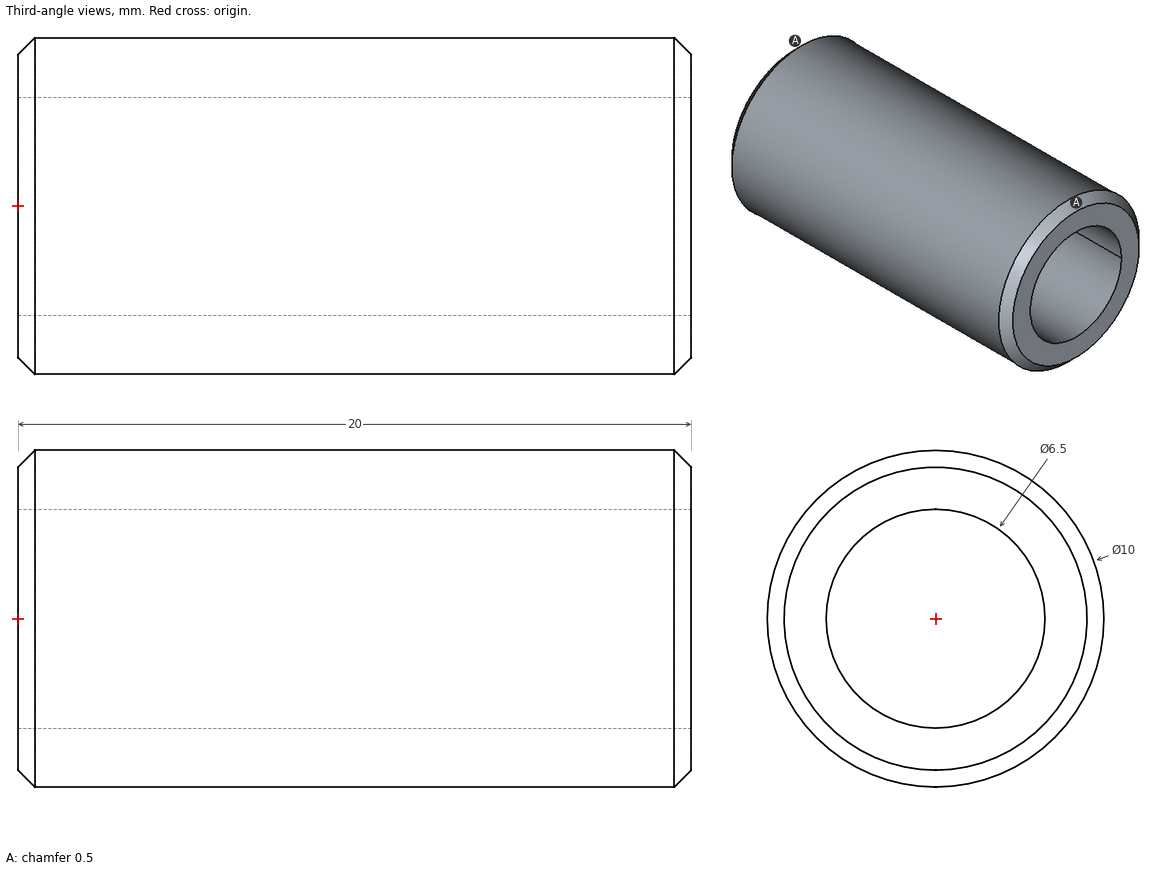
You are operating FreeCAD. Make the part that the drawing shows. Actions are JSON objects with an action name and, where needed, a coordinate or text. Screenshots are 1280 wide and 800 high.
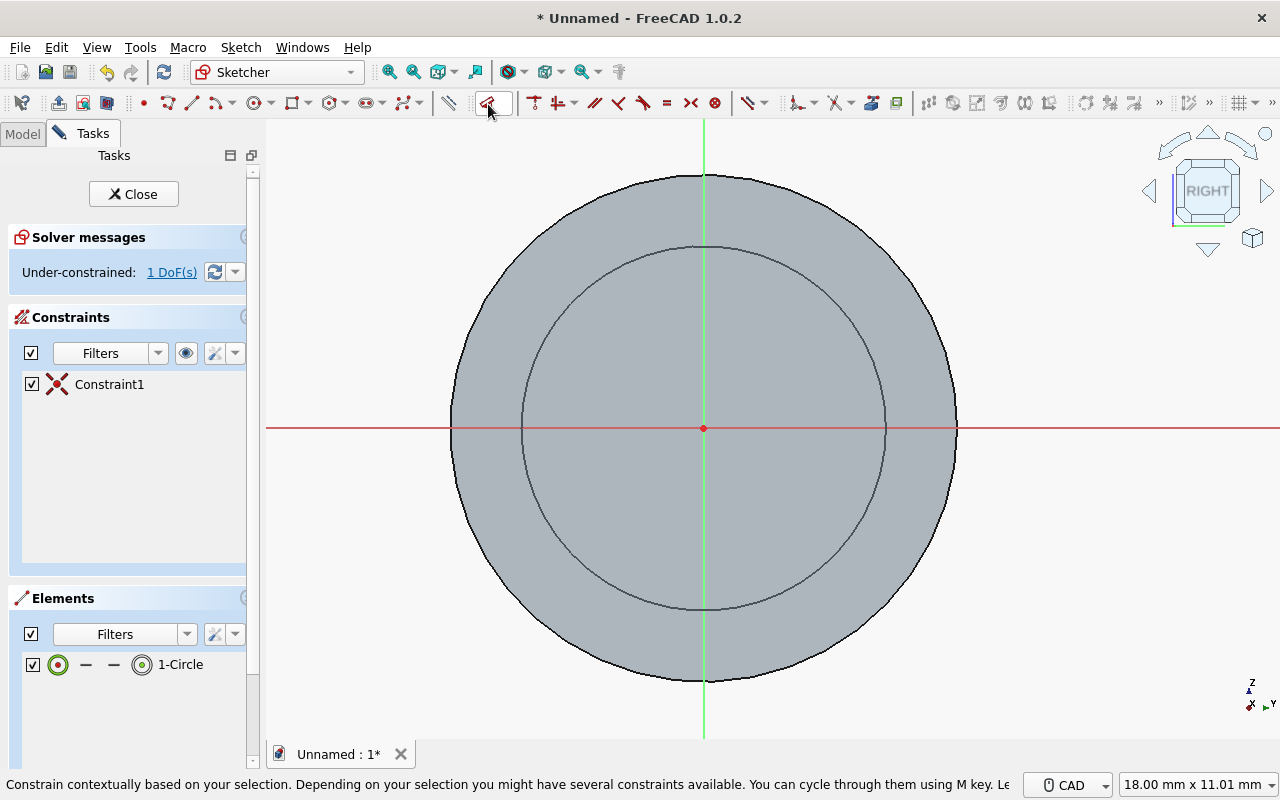
{"action": "left_click", "coordinate": [832, 299]}
{"action": "left_click", "coordinate": [855, 276]}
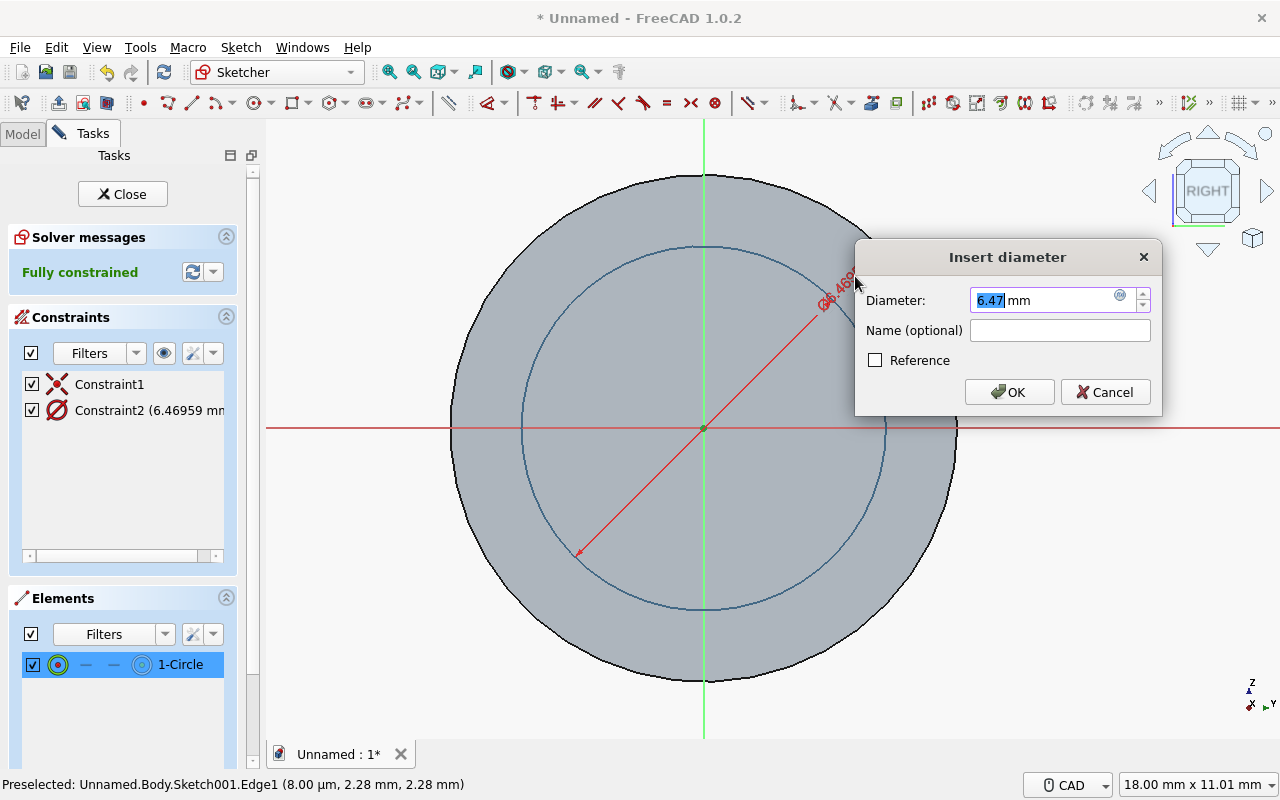
{"action": "type", "text": "6.5"}
{"action": "key", "text": "Return"}
{"action": "key", "text": "Escape"}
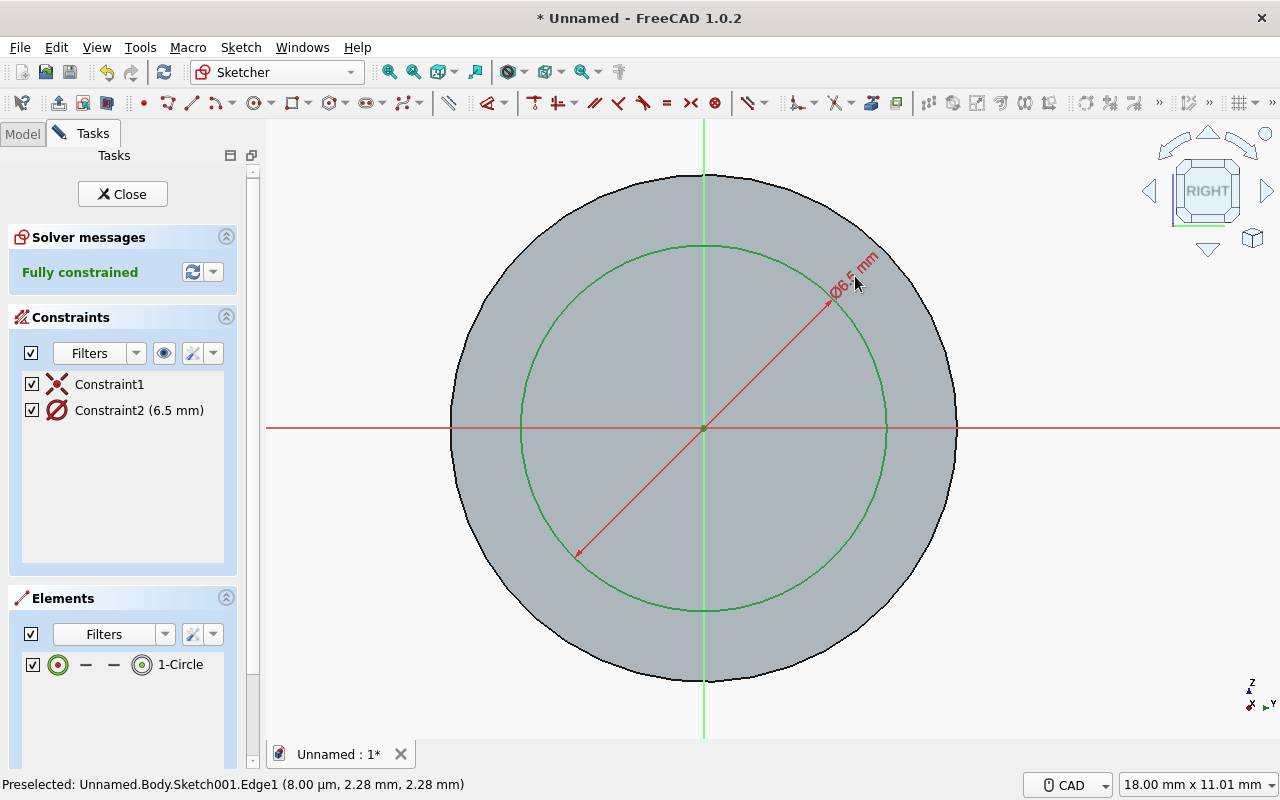
{"action": "left_click", "coordinate": [123, 194]}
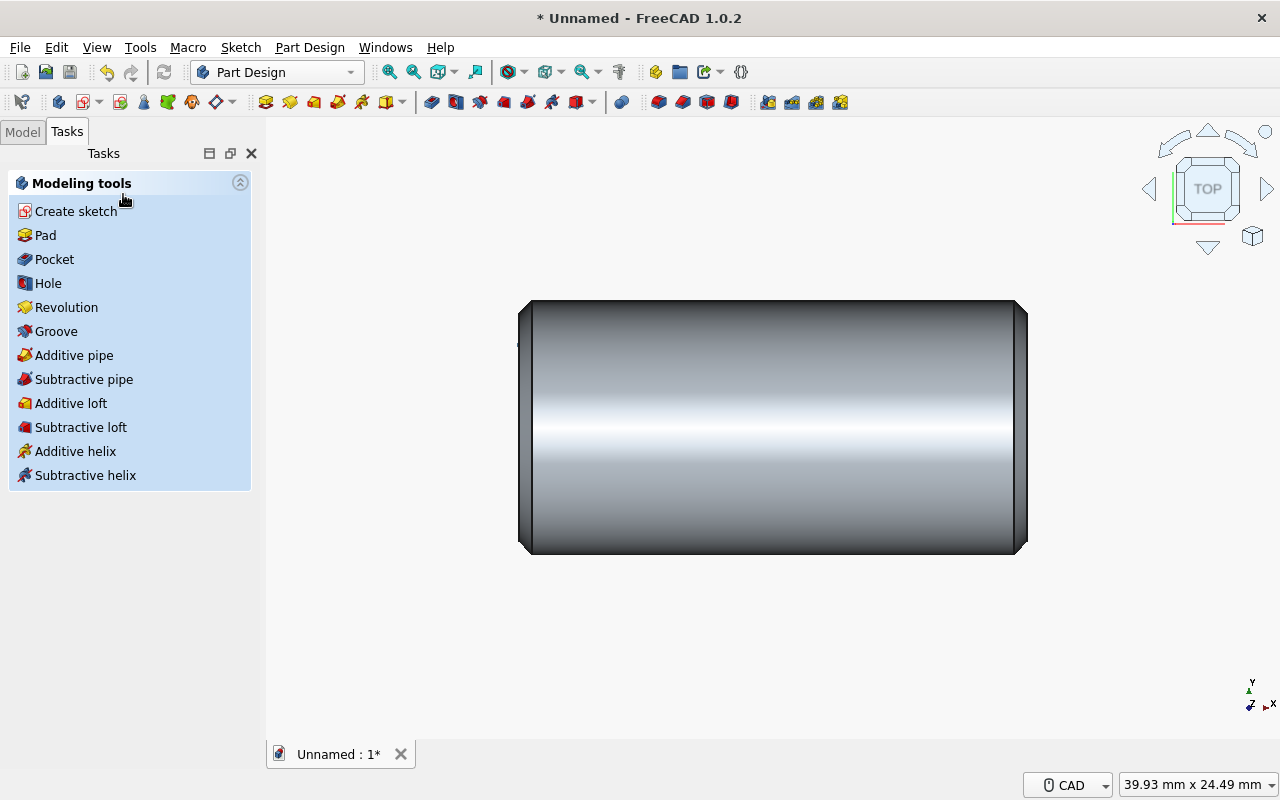
{"action": "left_click", "coordinate": [432, 102]}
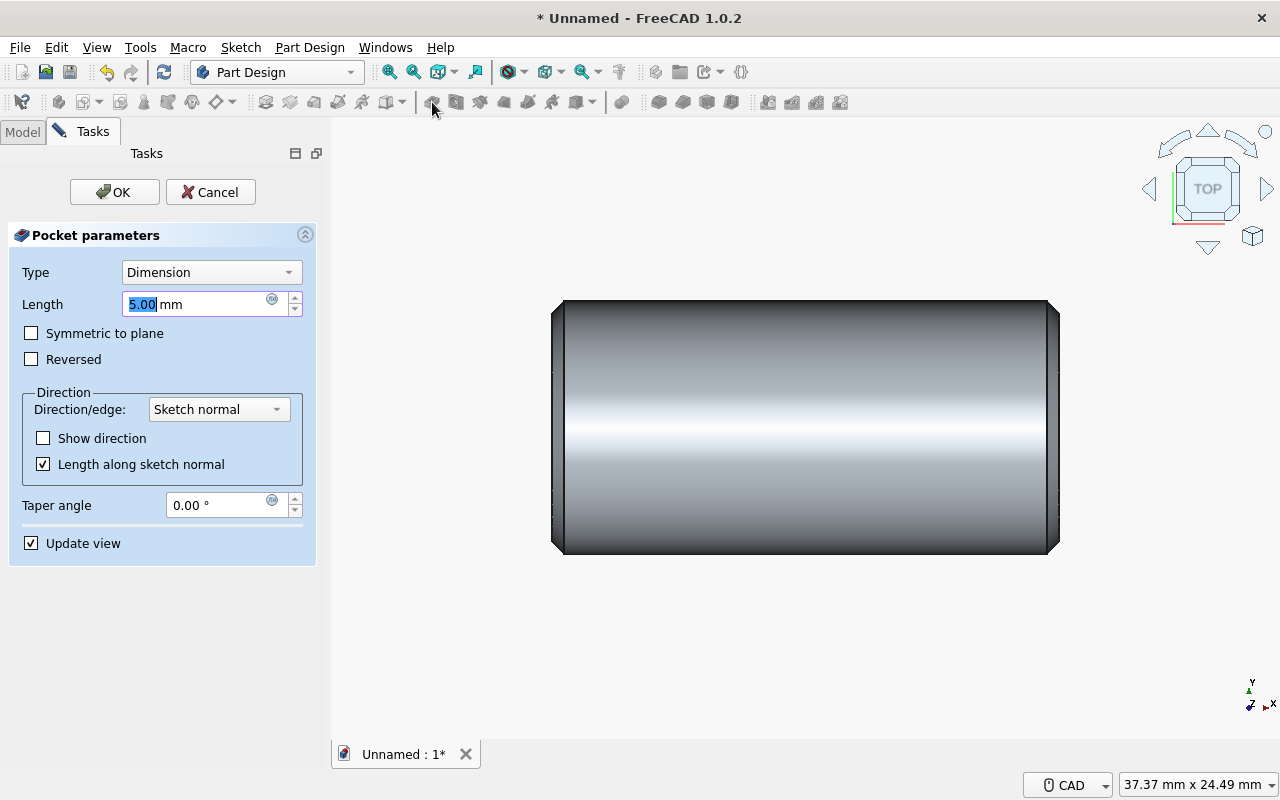
{"action": "left_click", "coordinate": [212, 272]}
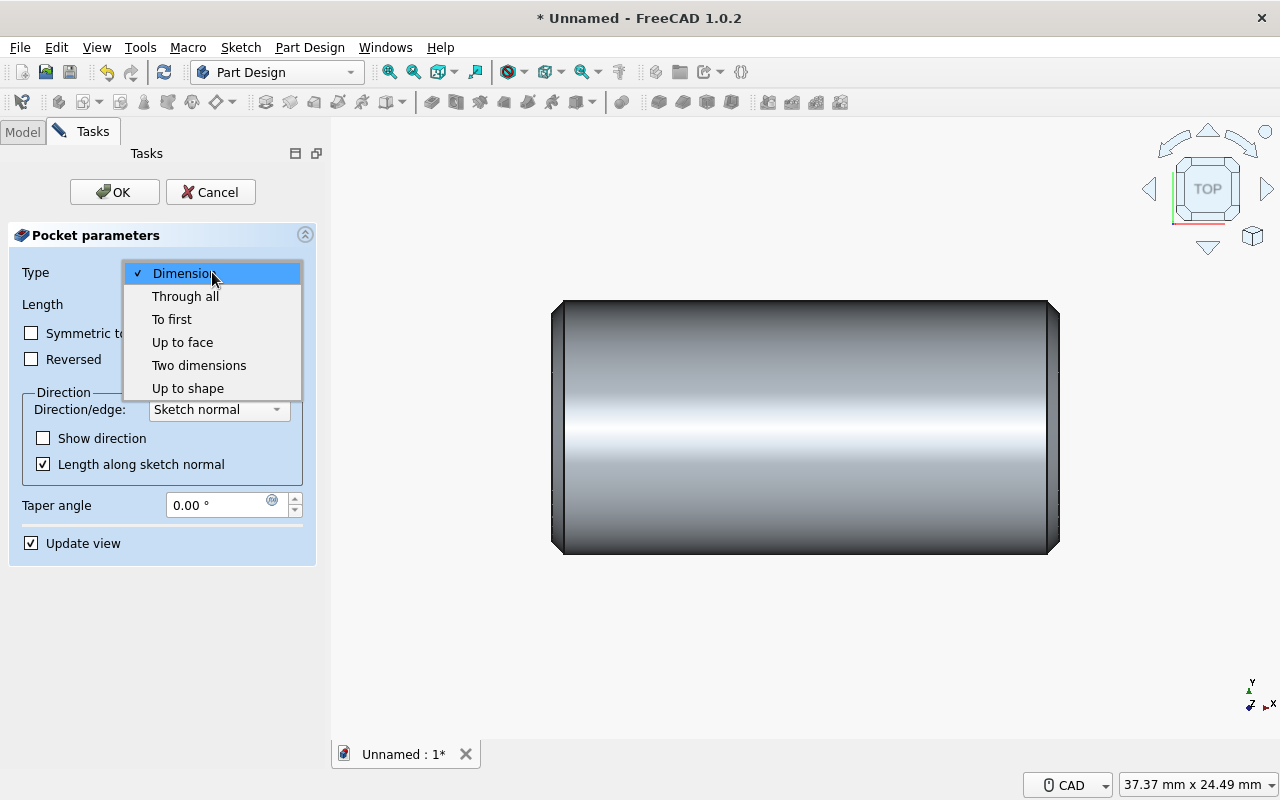
{"action": "left_click", "coordinate": [212, 296]}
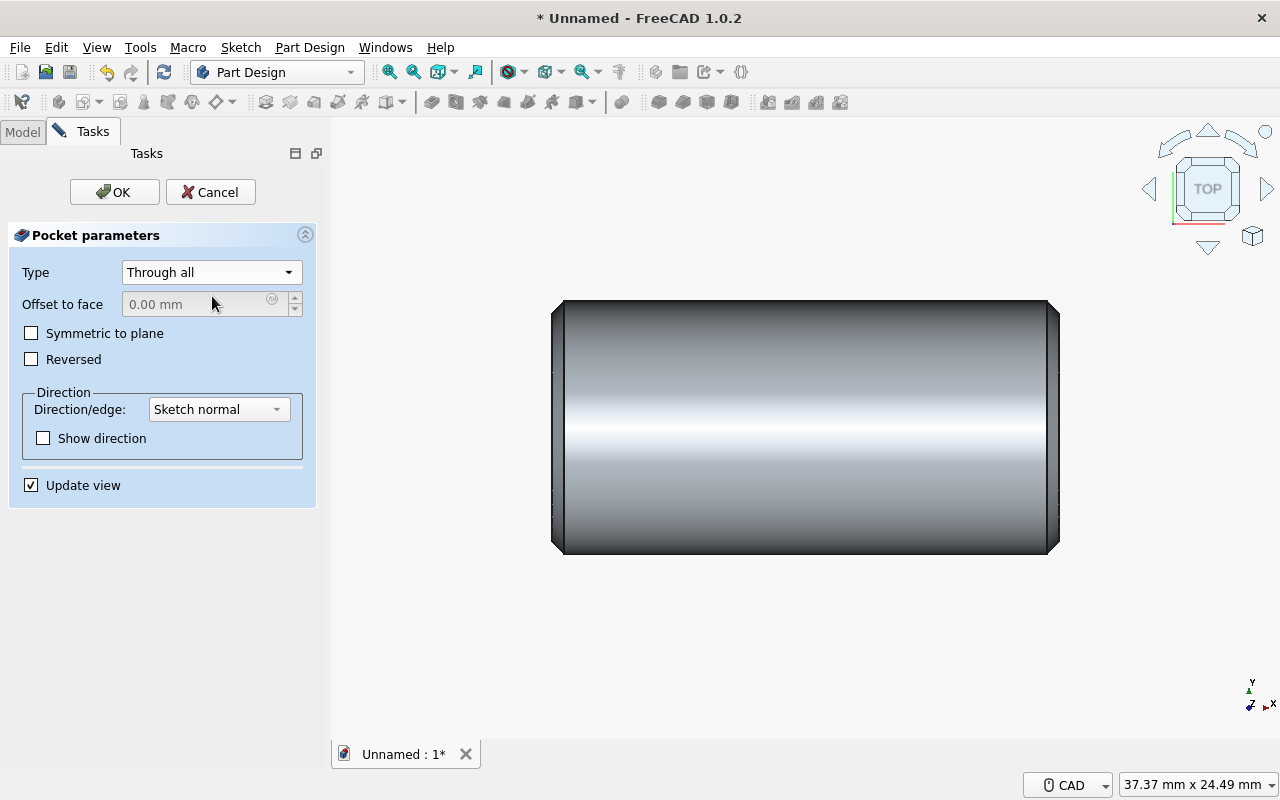
{"action": "left_click", "coordinate": [30, 359]}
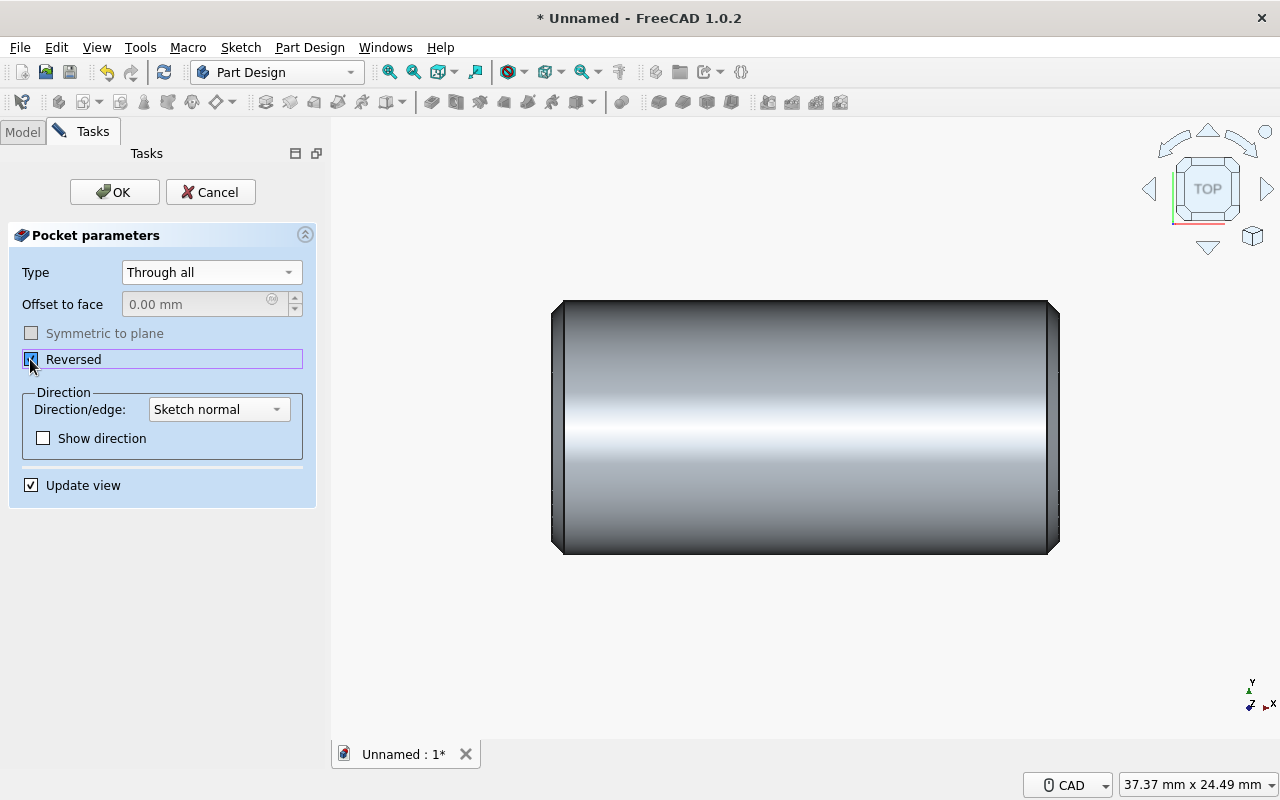
{"action": "left_click", "coordinate": [115, 192]}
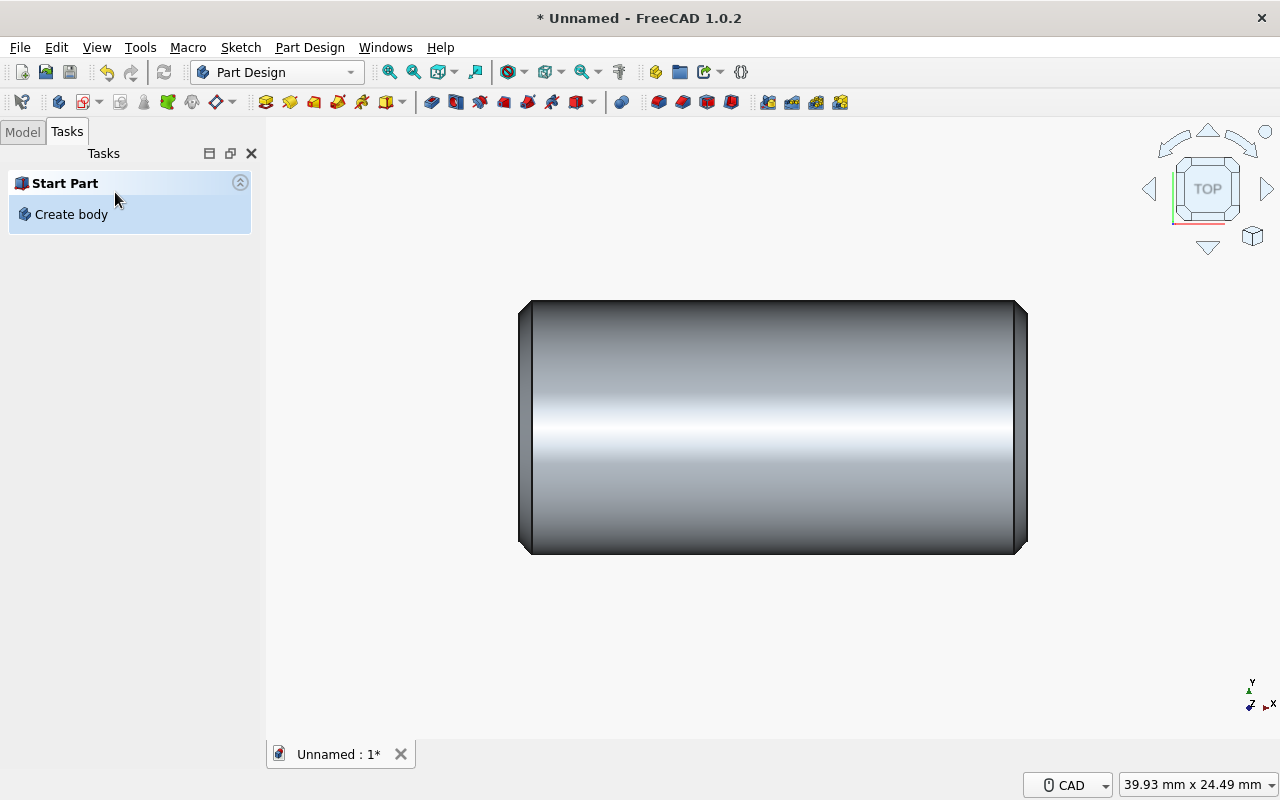
{"action": "key", "text": "0"}